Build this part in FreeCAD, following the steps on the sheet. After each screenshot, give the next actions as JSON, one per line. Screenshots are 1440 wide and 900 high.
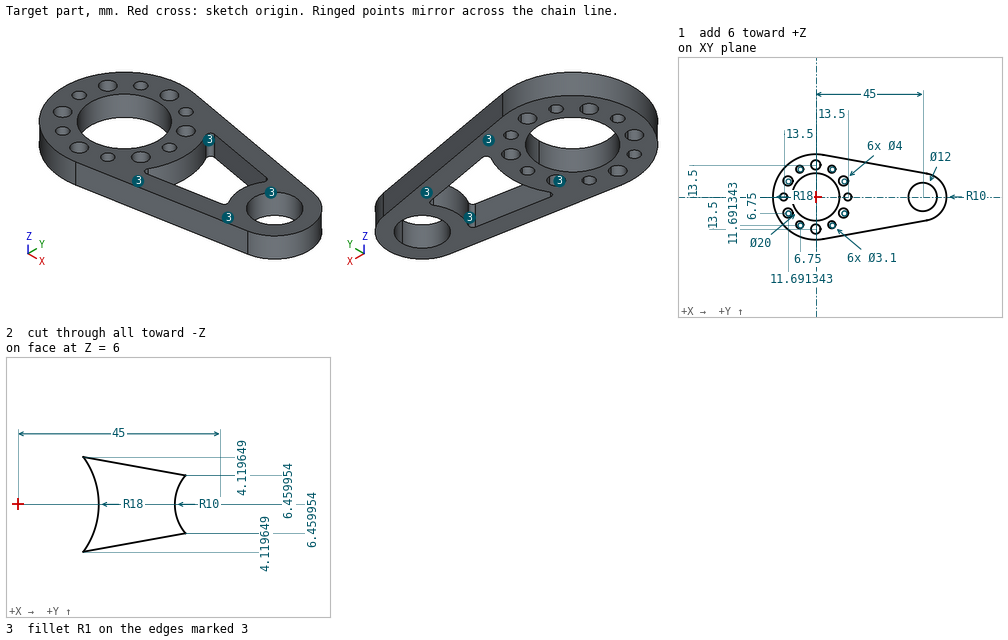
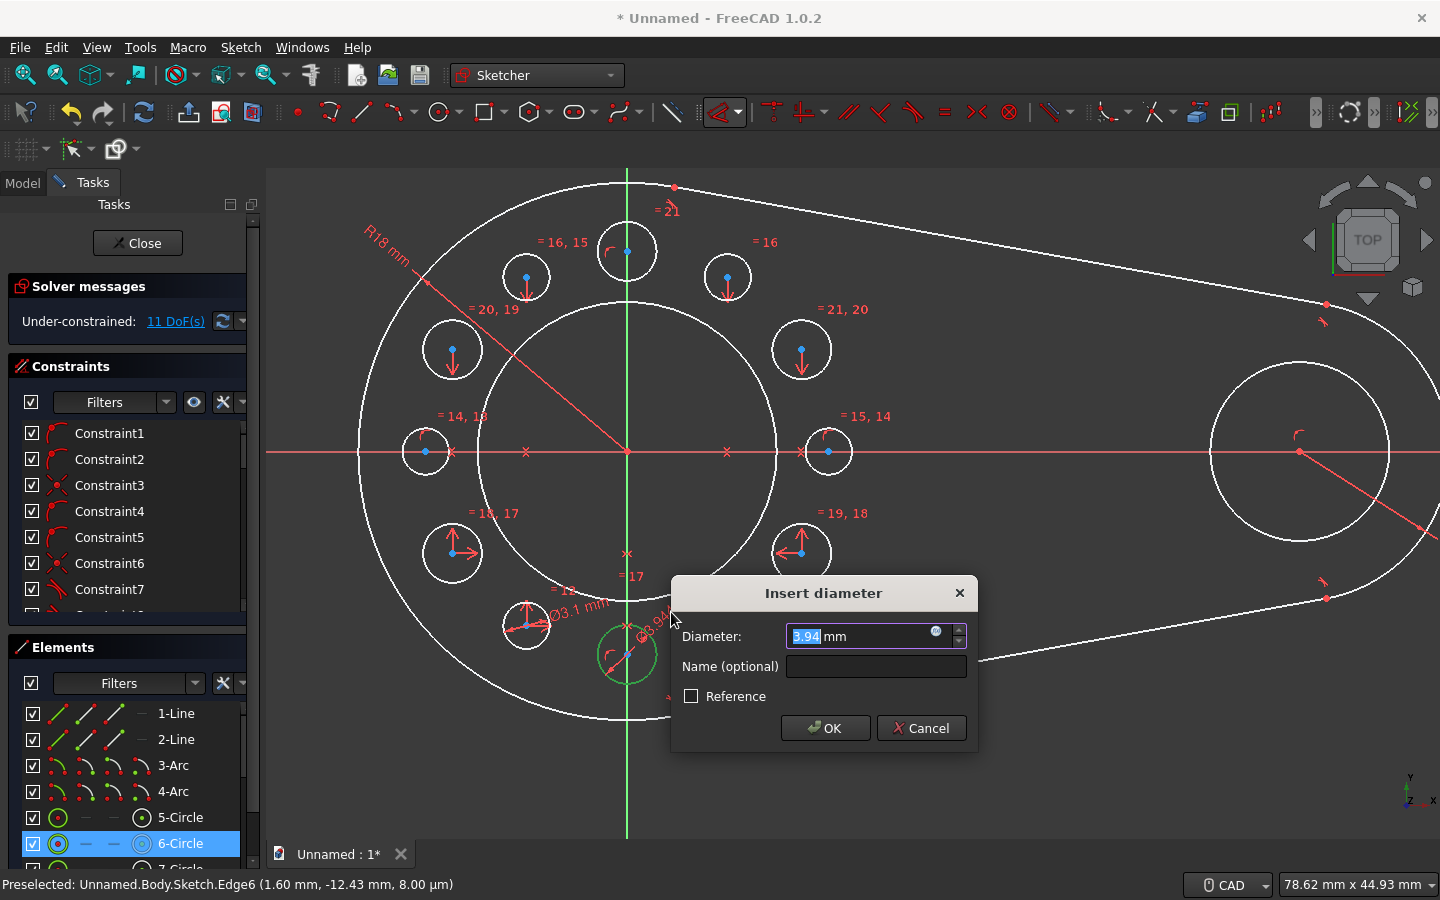
{"action": "type", "text": "4"}
{"action": "key", "text": "Return"}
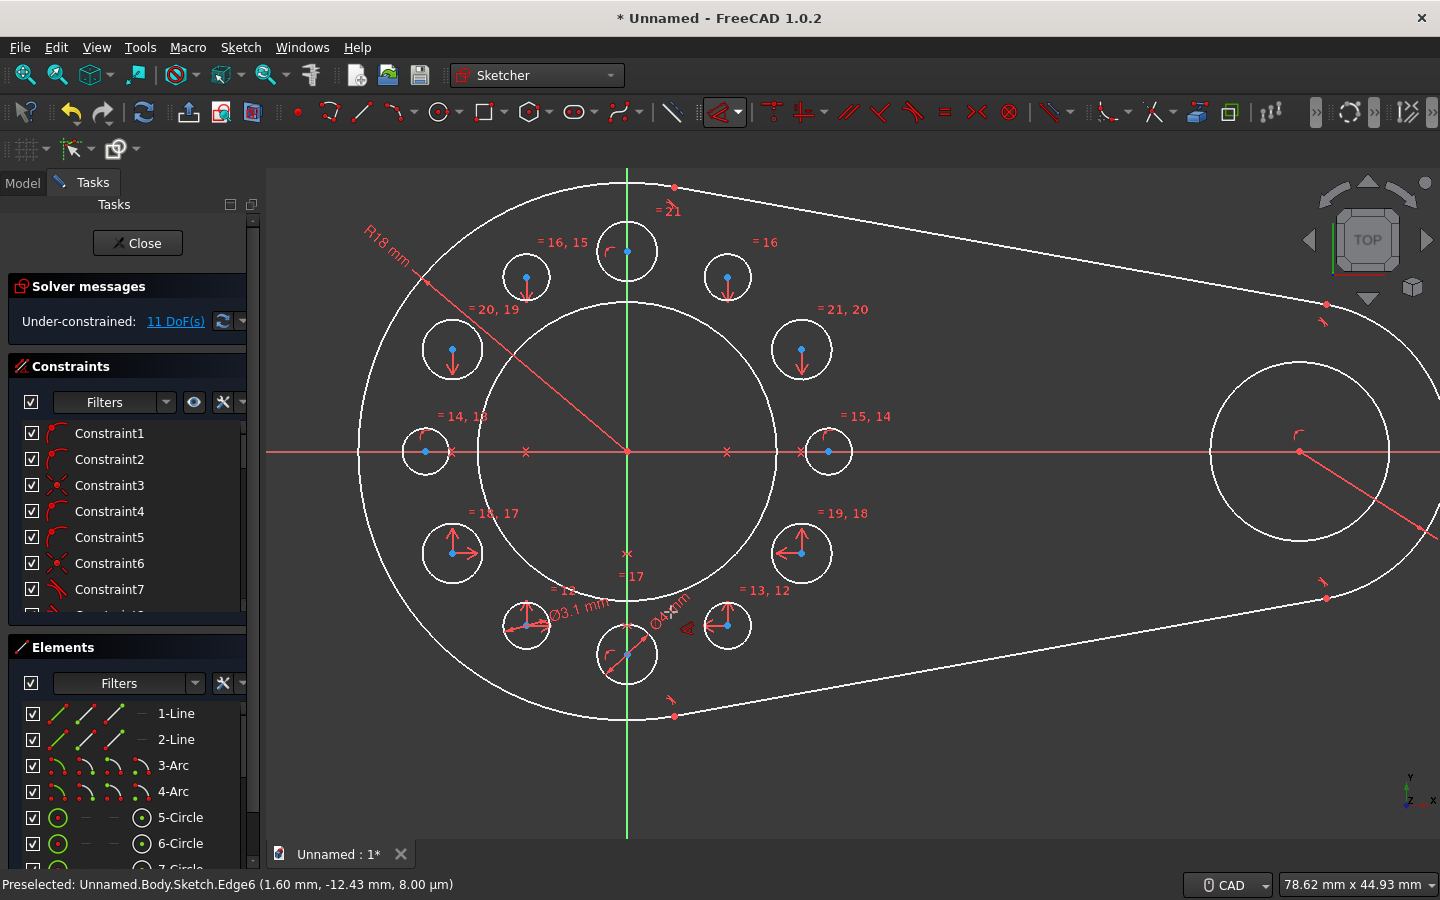
{"action": "left_click", "coordinate": [733, 345]}
{"action": "left_click", "coordinate": [756, 322]}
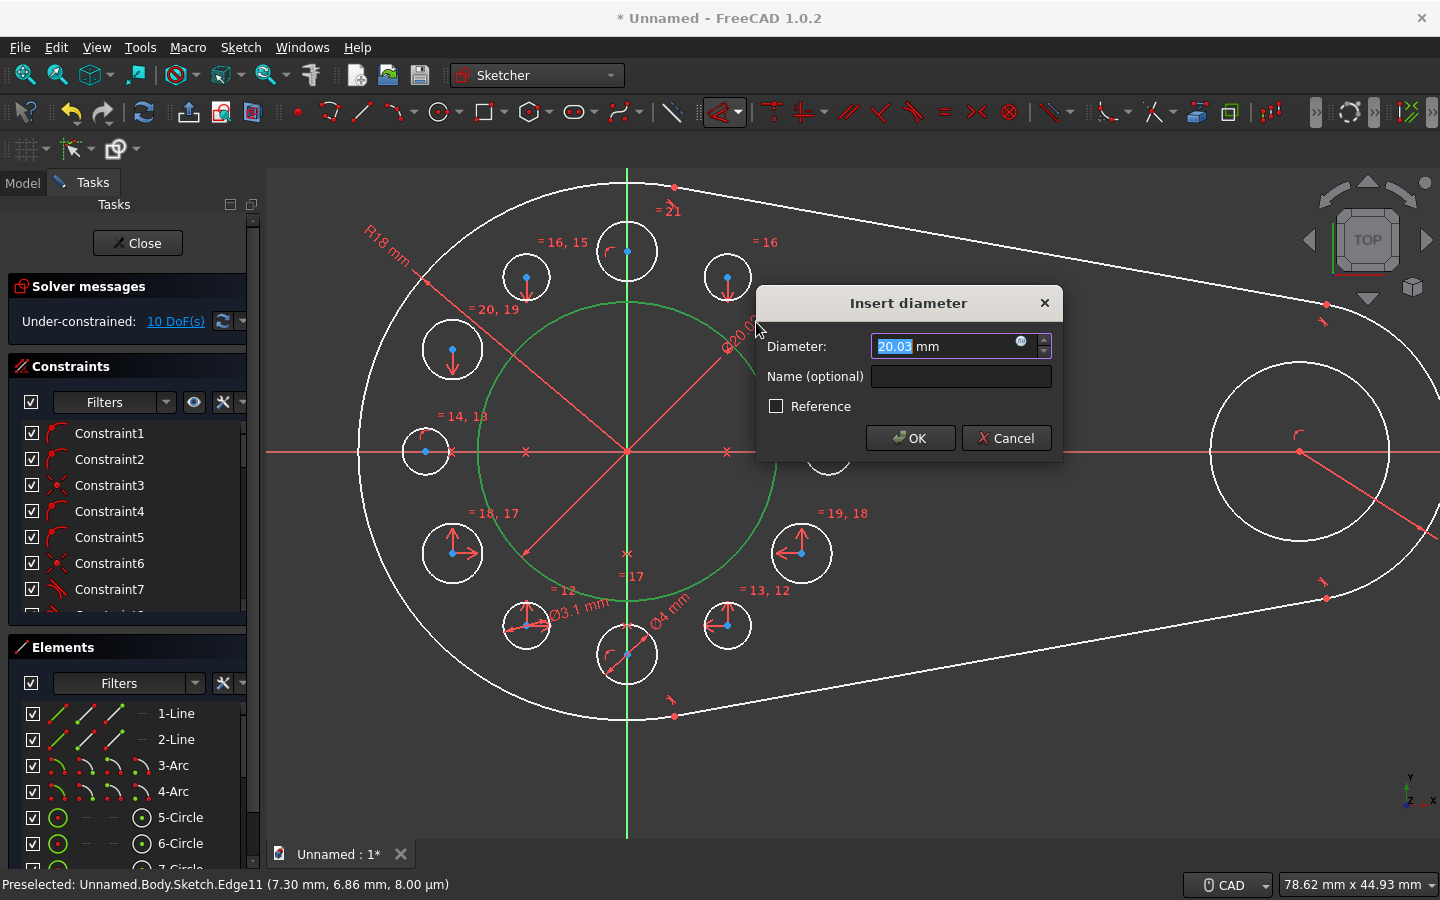
{"action": "type", "text": "20"}
{"action": "key", "text": "Return"}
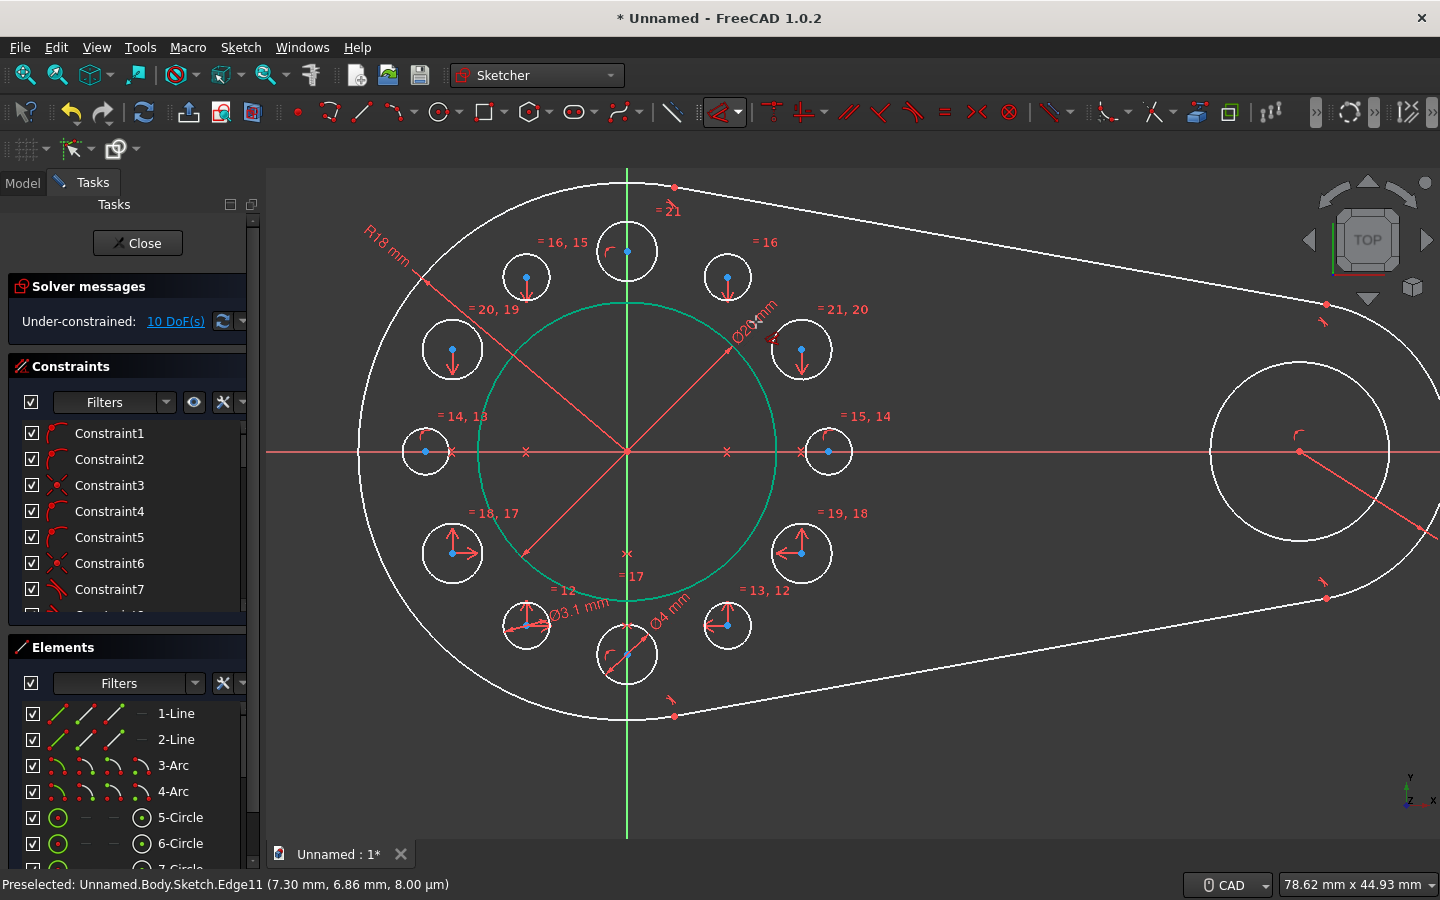
{"action": "left_click", "coordinate": [1236, 388]}
{"action": "left_click", "coordinate": [1213, 365]}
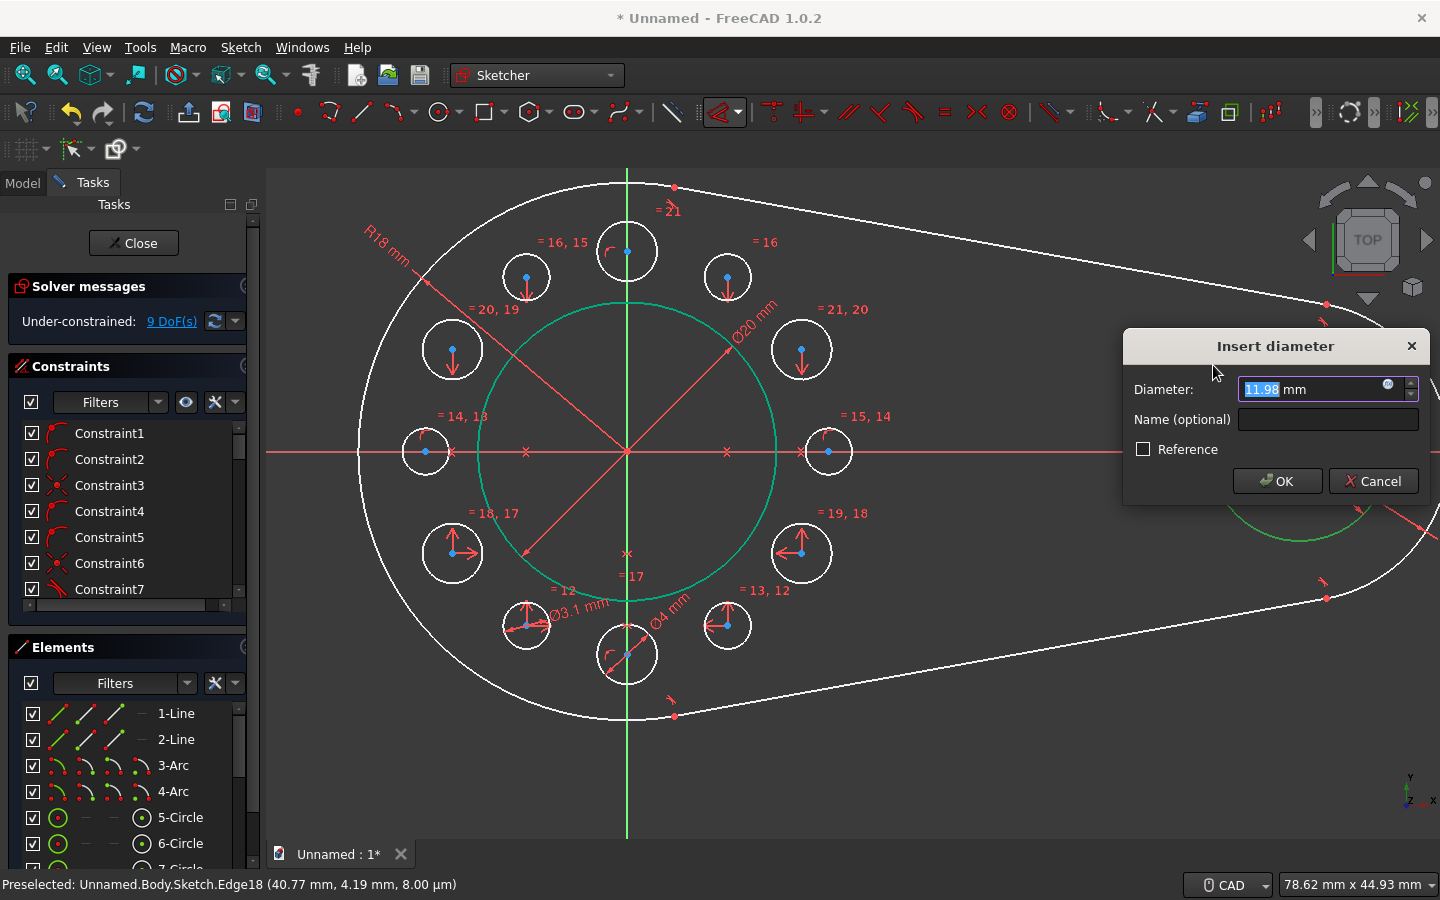
{"action": "type", "text": "12"}
{"action": "key", "text": "Return"}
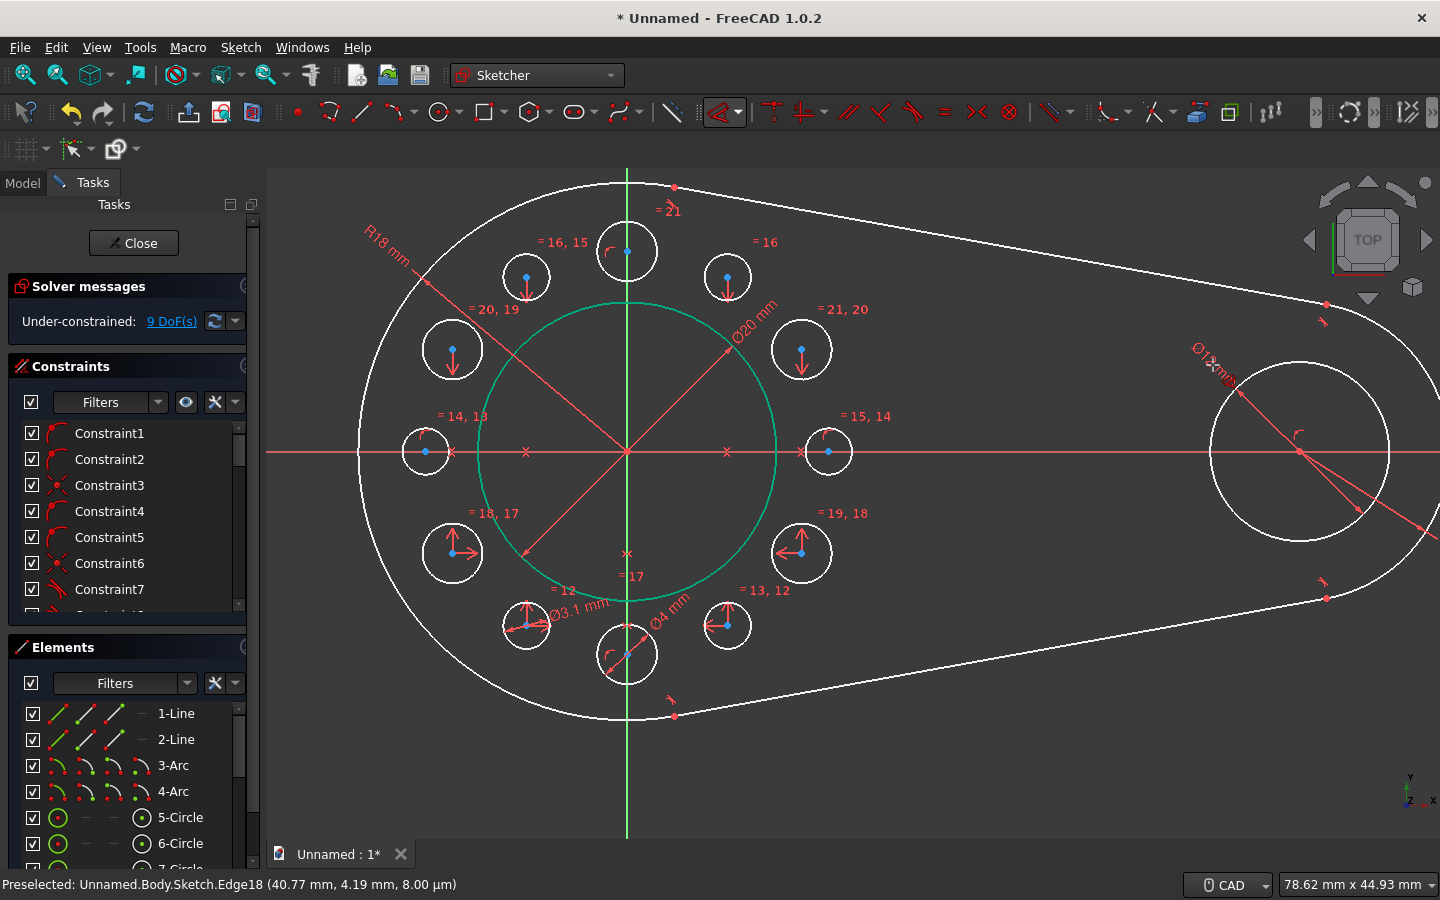
{"action": "scroll", "coordinate": [543, 609], "scroll_direction": "down", "scroll_amount": 2}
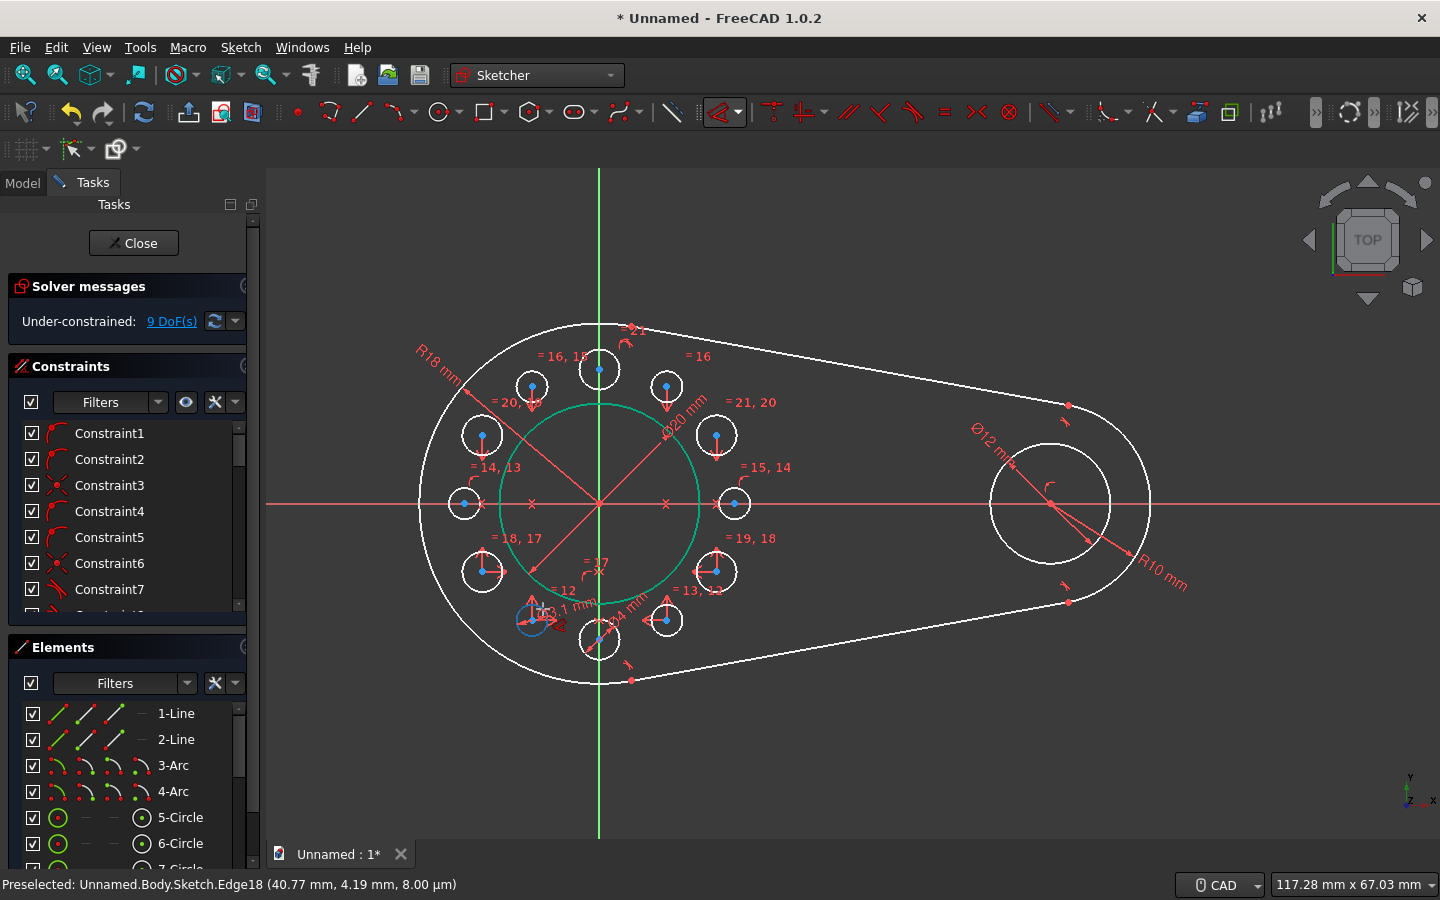
{"action": "left_click", "coordinate": [1050, 504]}
{"action": "left_click", "coordinate": [825, 538]}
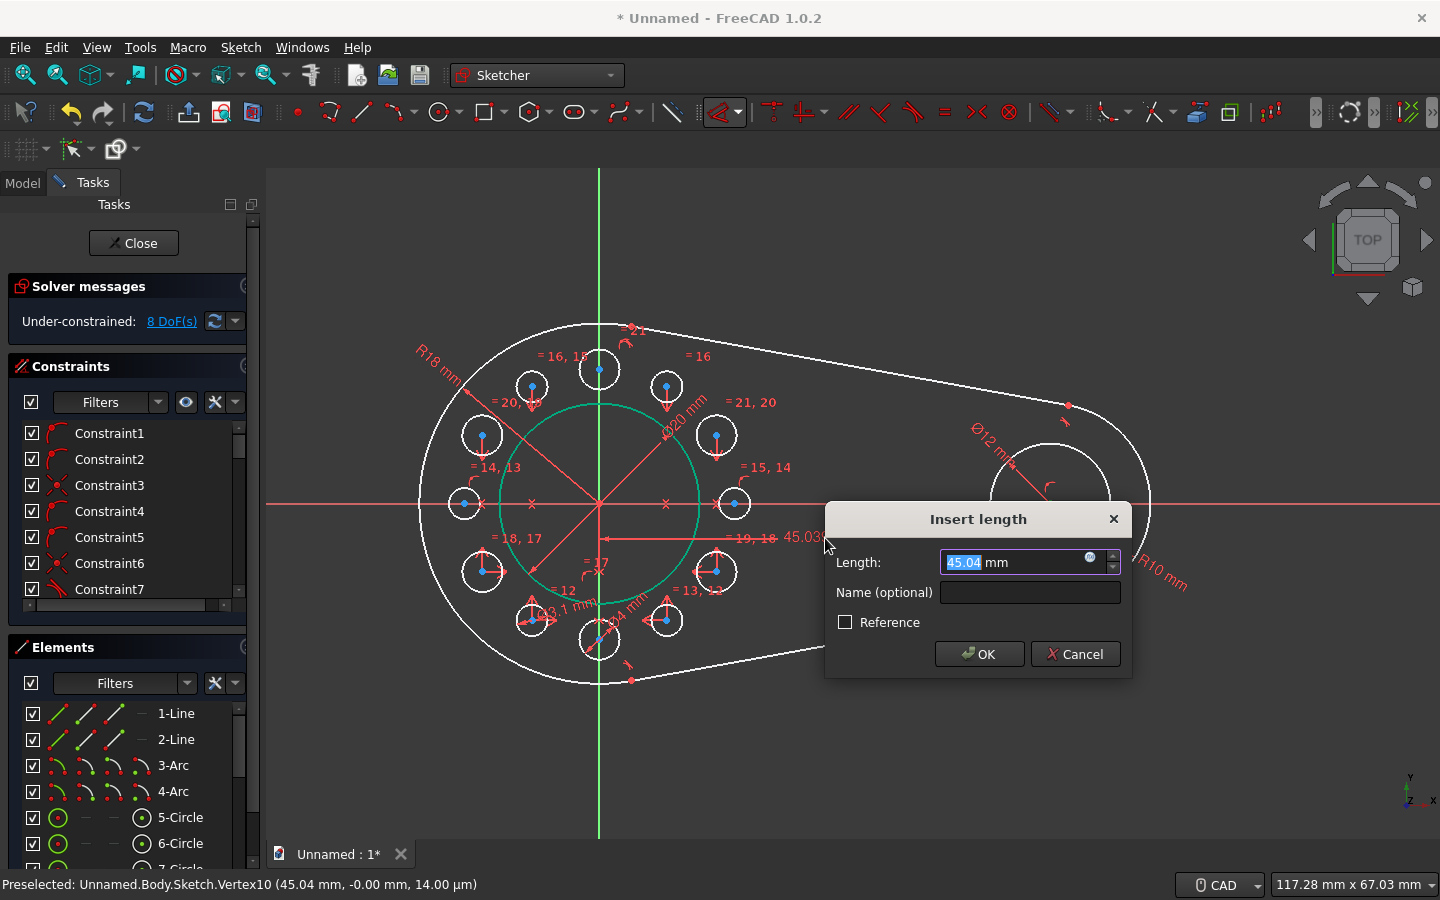
{"action": "type", "text": "45"}
{"action": "key", "text": "Return"}